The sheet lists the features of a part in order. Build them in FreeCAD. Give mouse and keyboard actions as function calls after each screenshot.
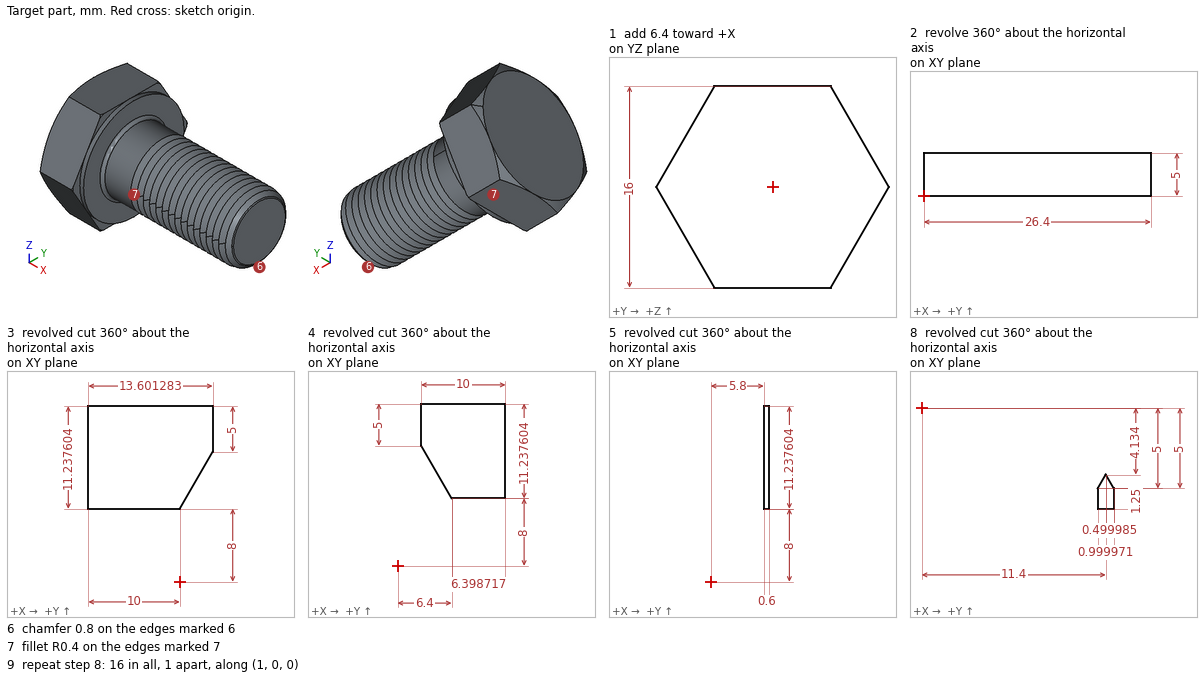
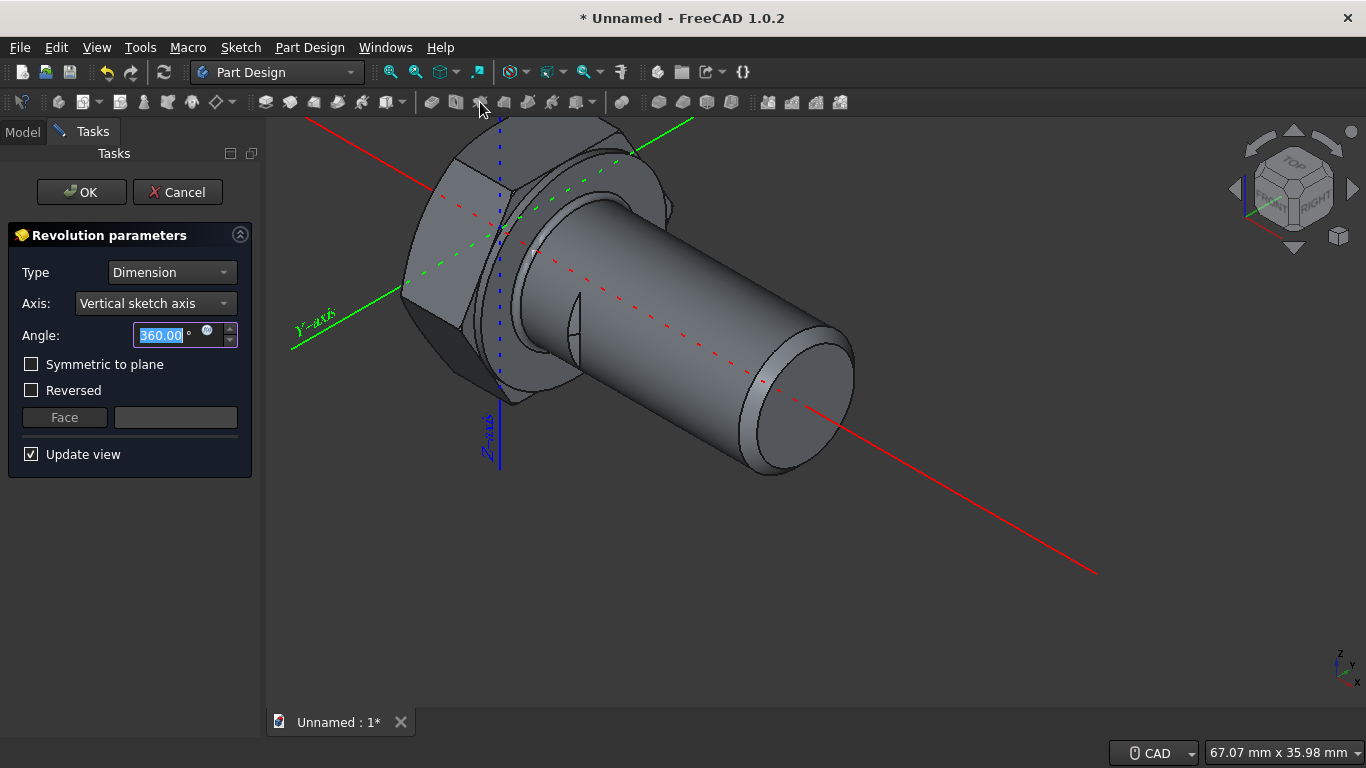
click(156, 304)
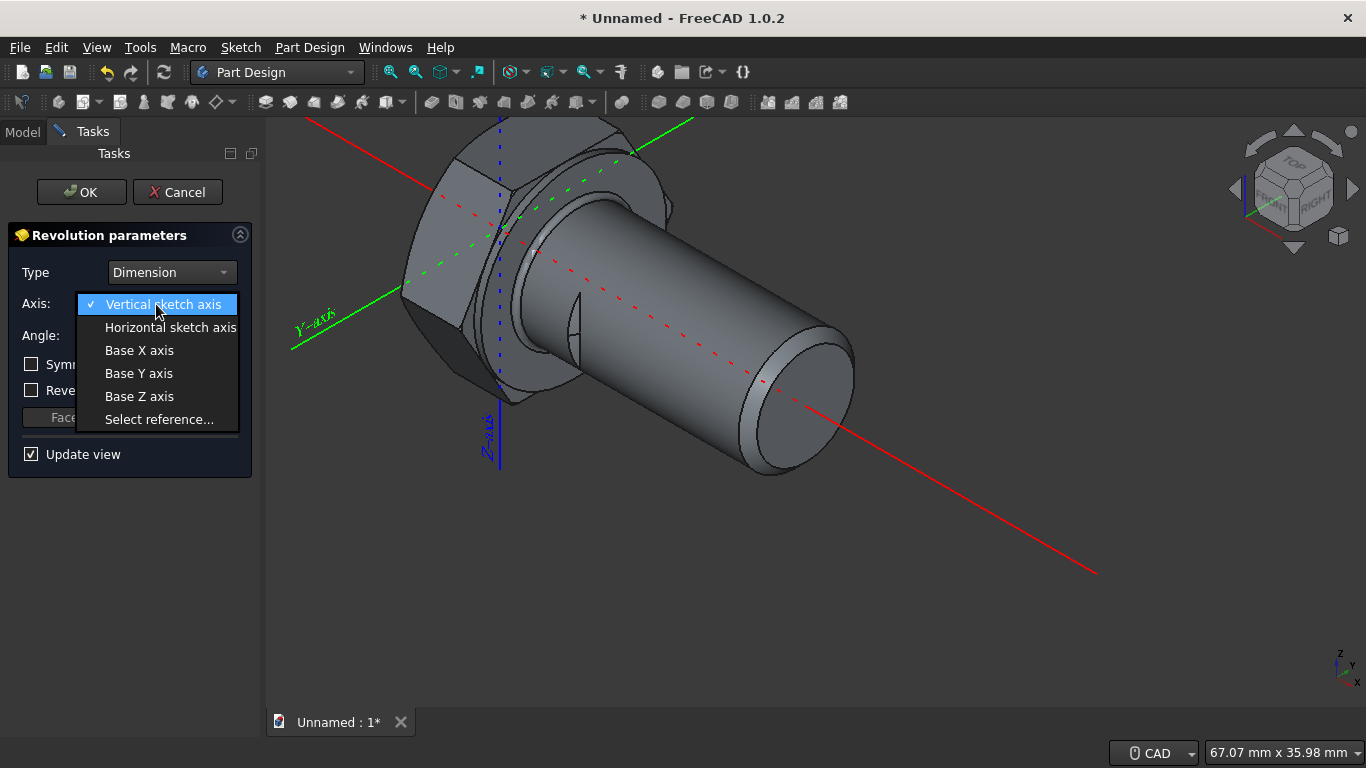
click(156, 328)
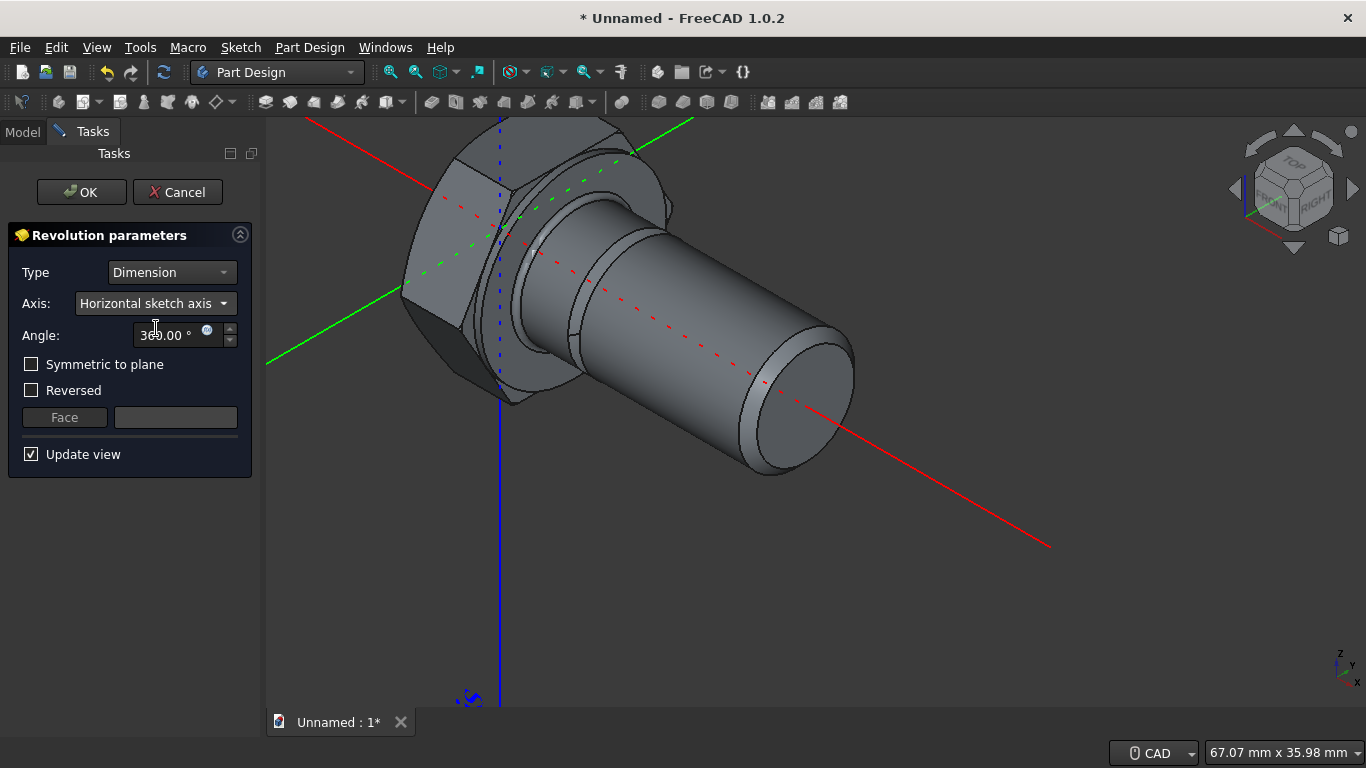
click(82, 192)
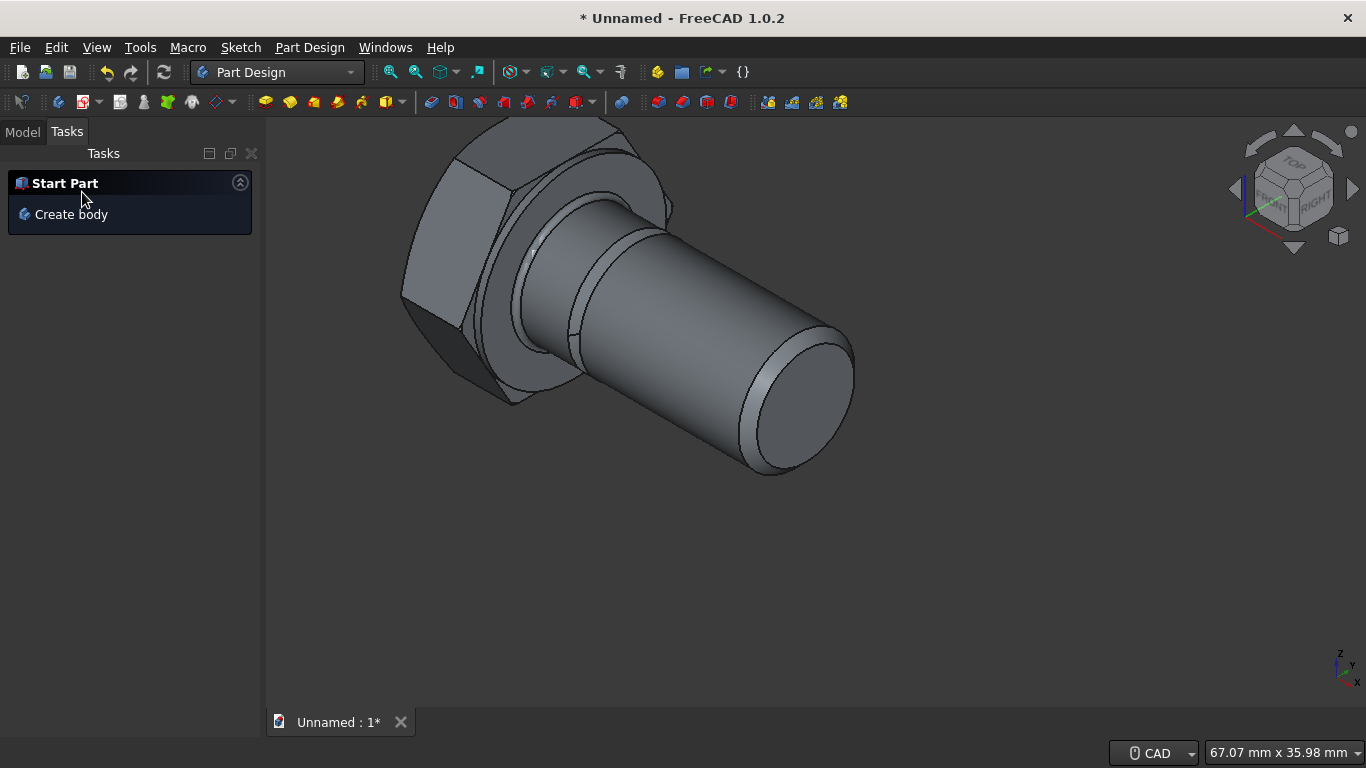
click(392, 72)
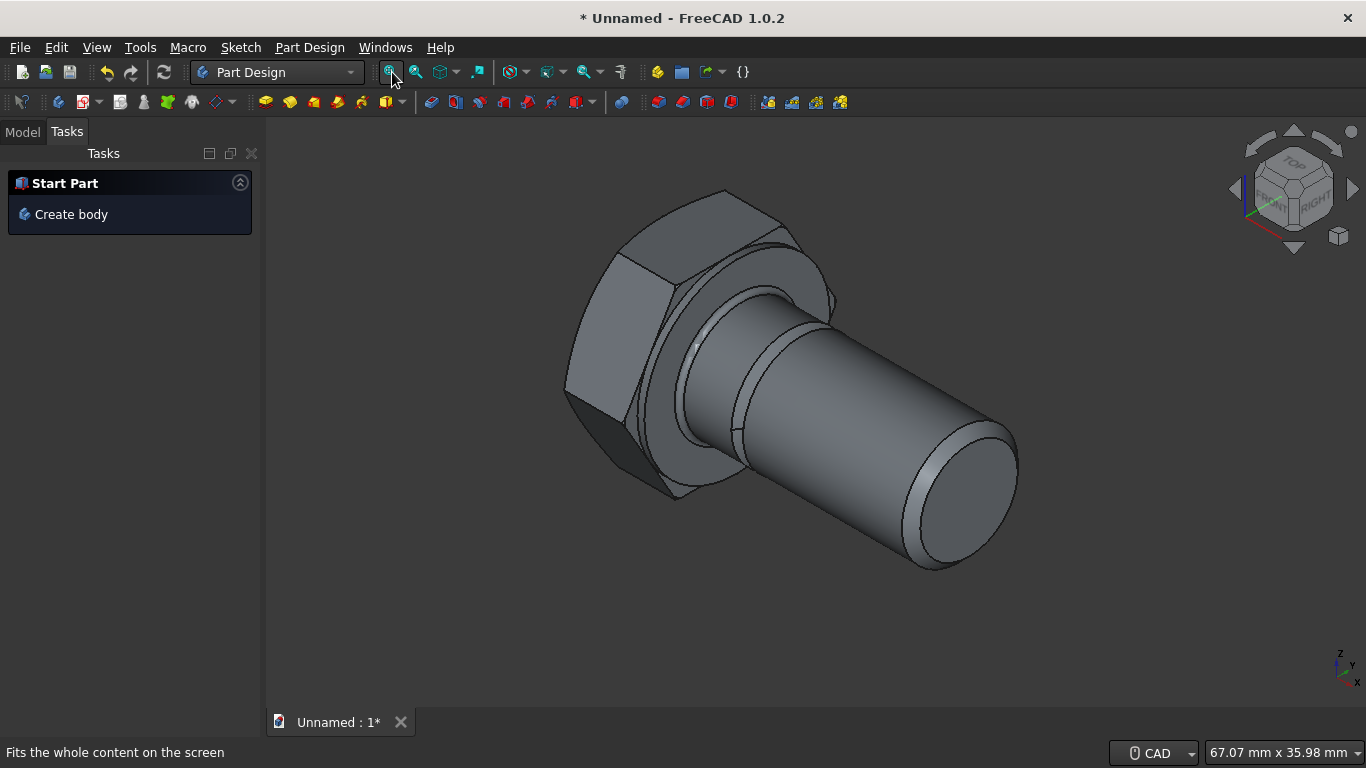
click(23, 131)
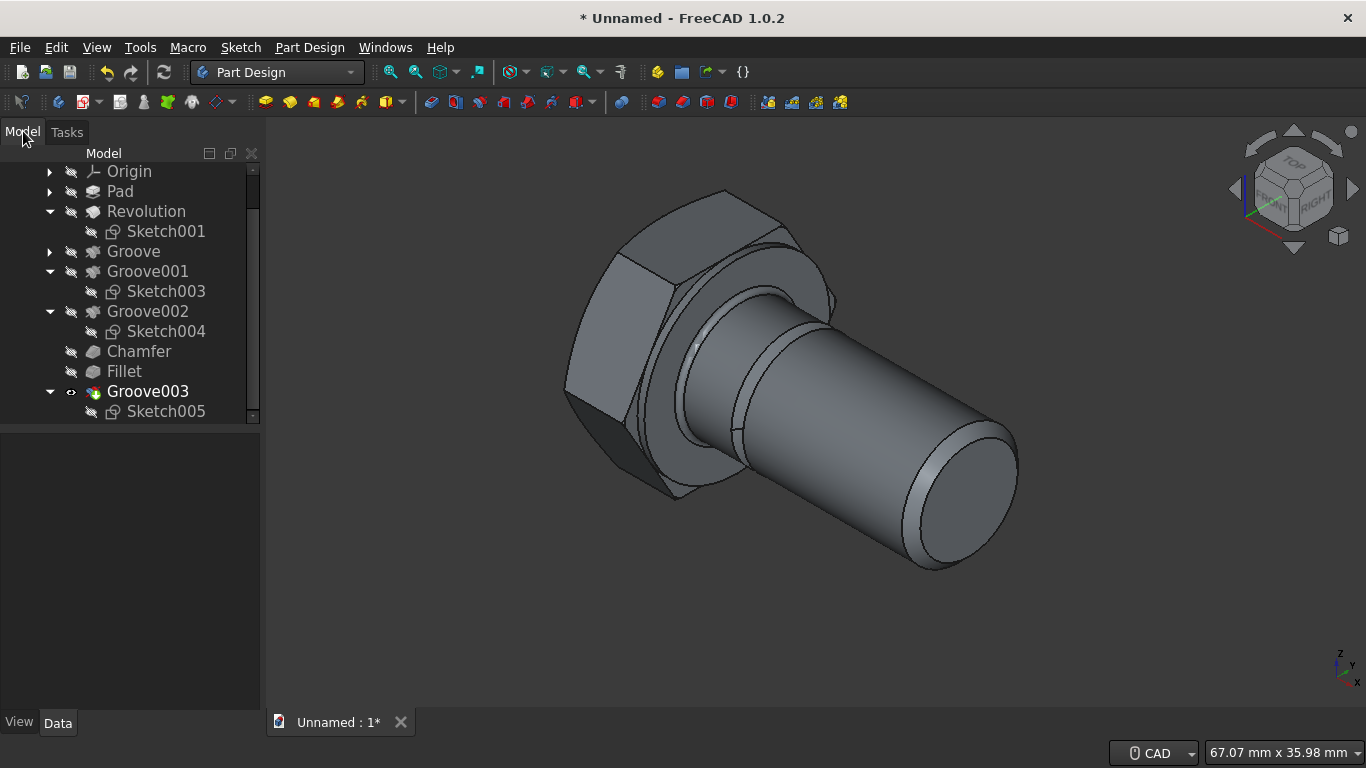
click(116, 392)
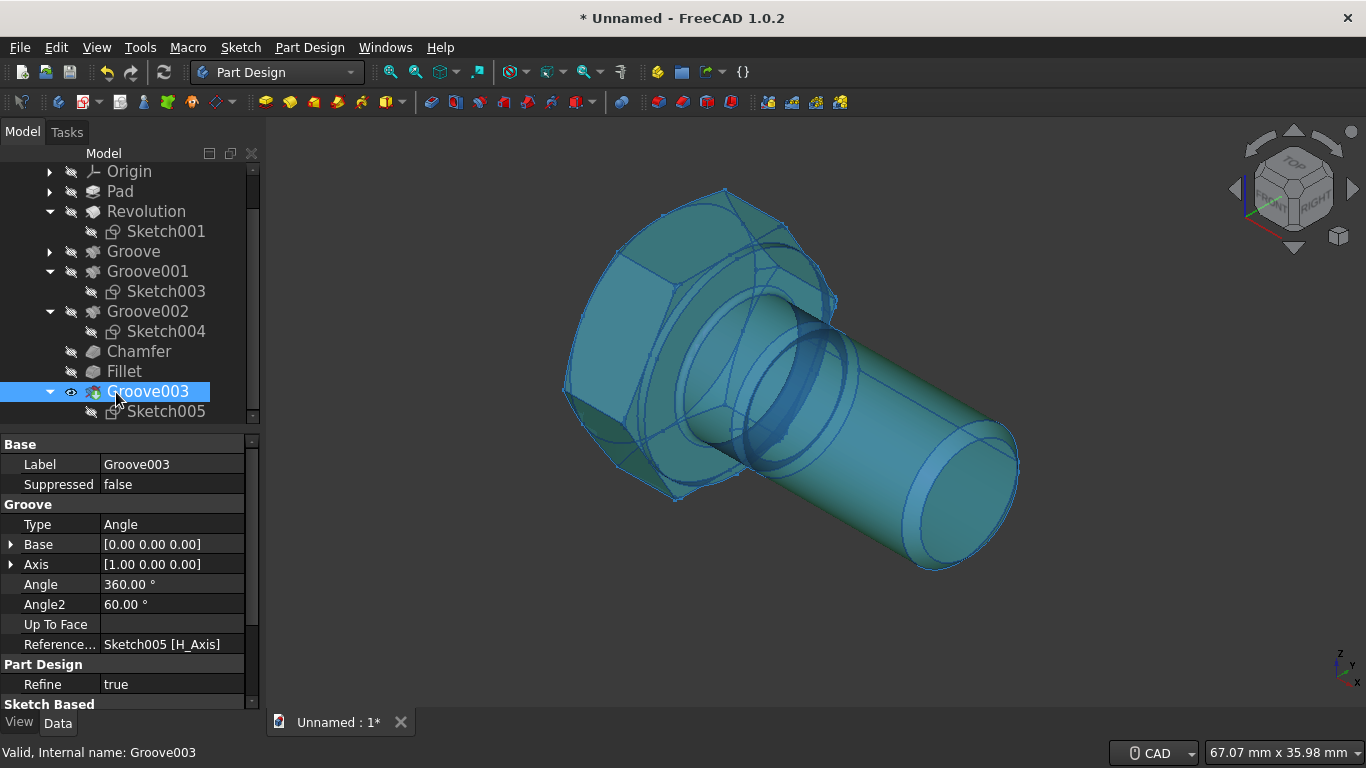
click(792, 102)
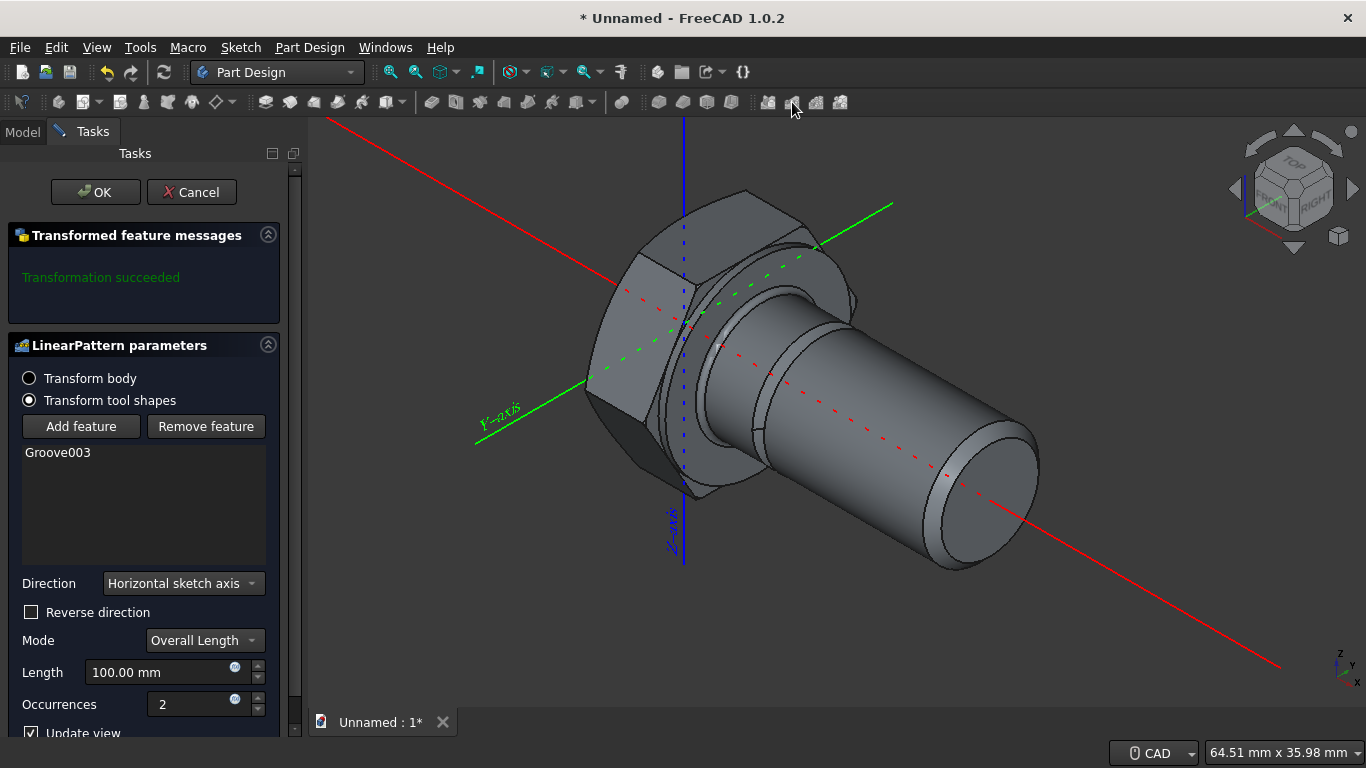
click(184, 584)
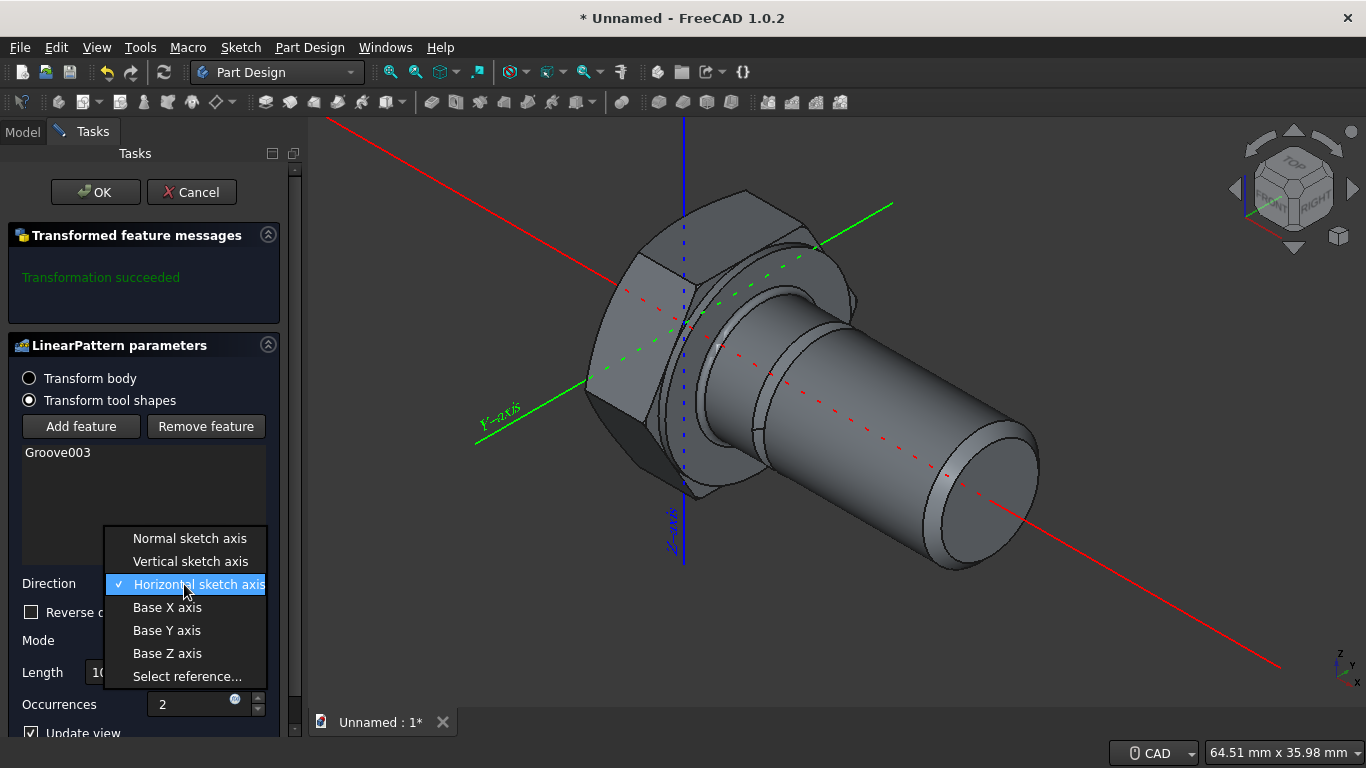
click(184, 608)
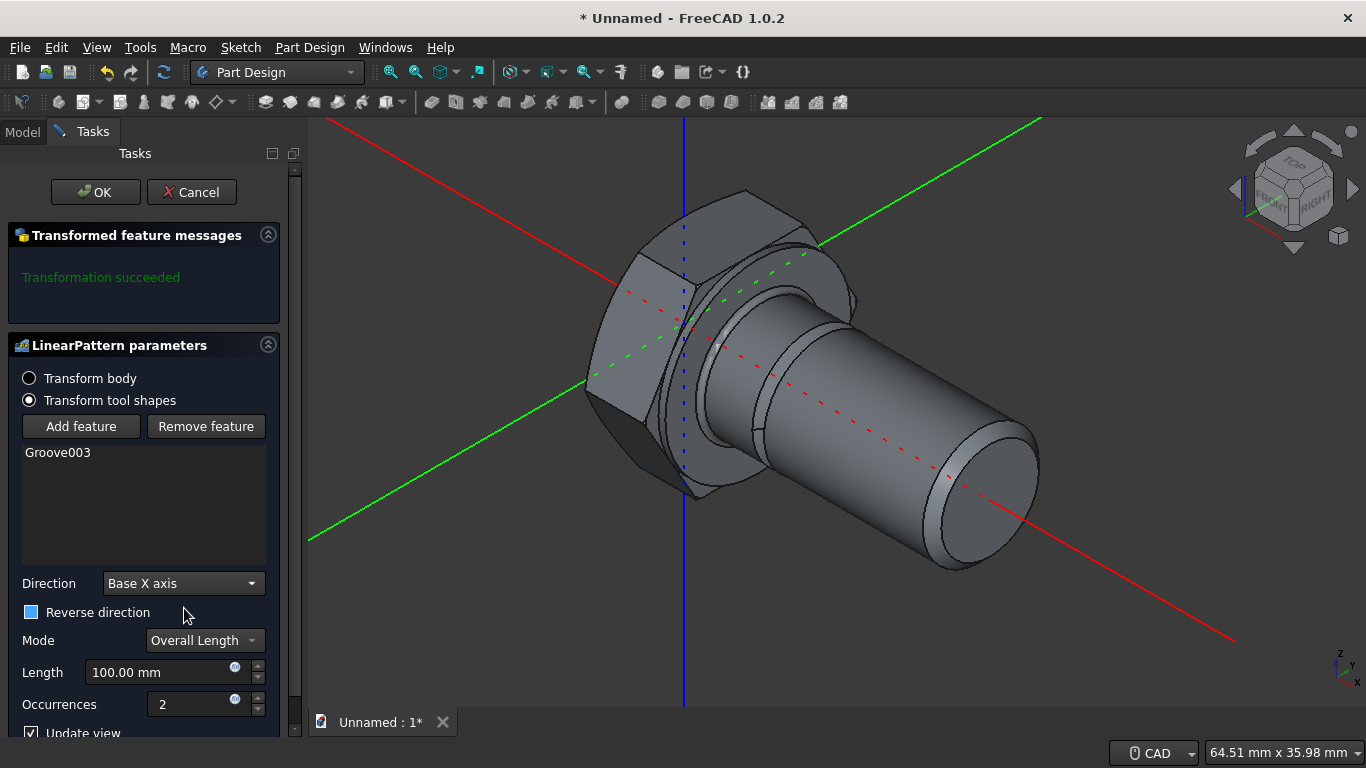
click(206, 640)